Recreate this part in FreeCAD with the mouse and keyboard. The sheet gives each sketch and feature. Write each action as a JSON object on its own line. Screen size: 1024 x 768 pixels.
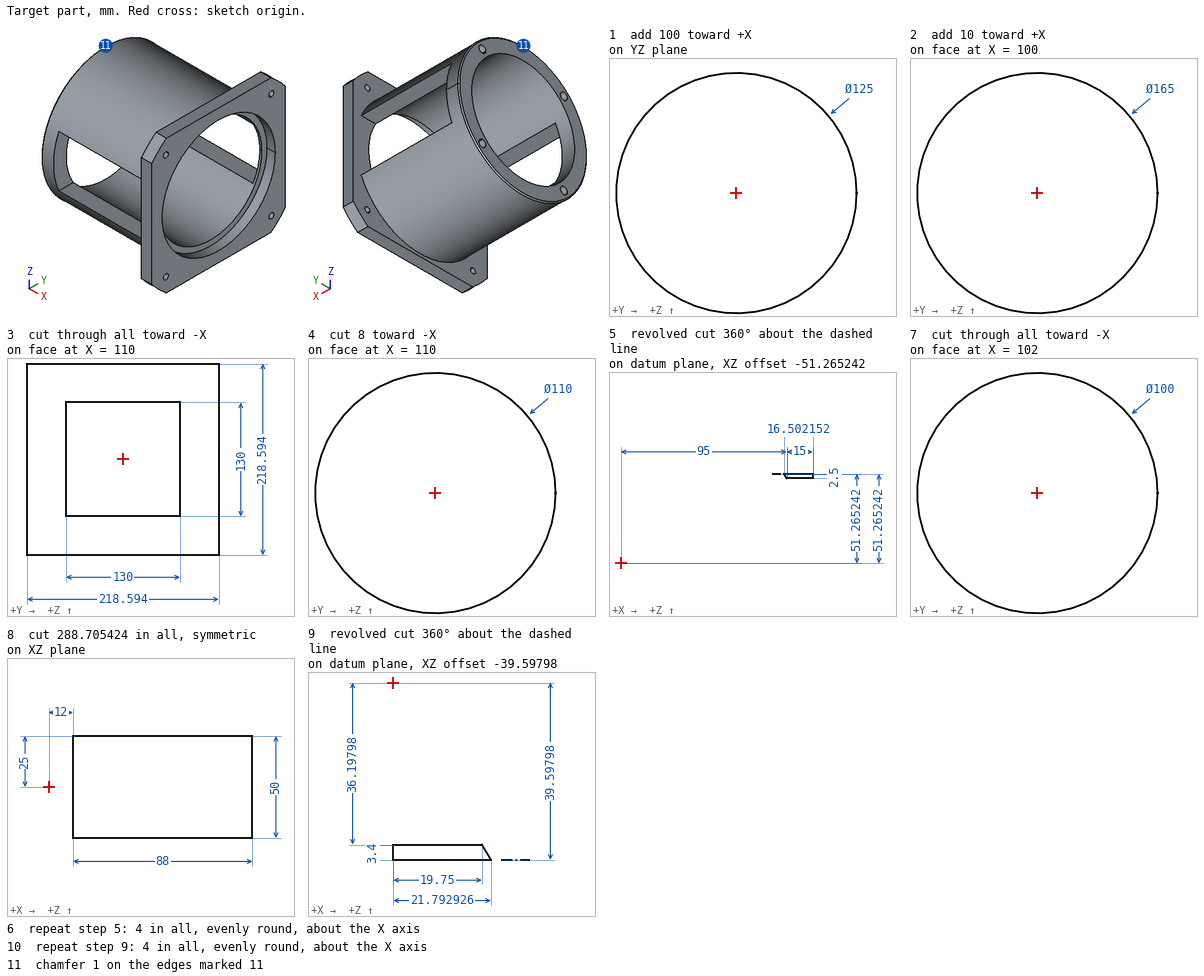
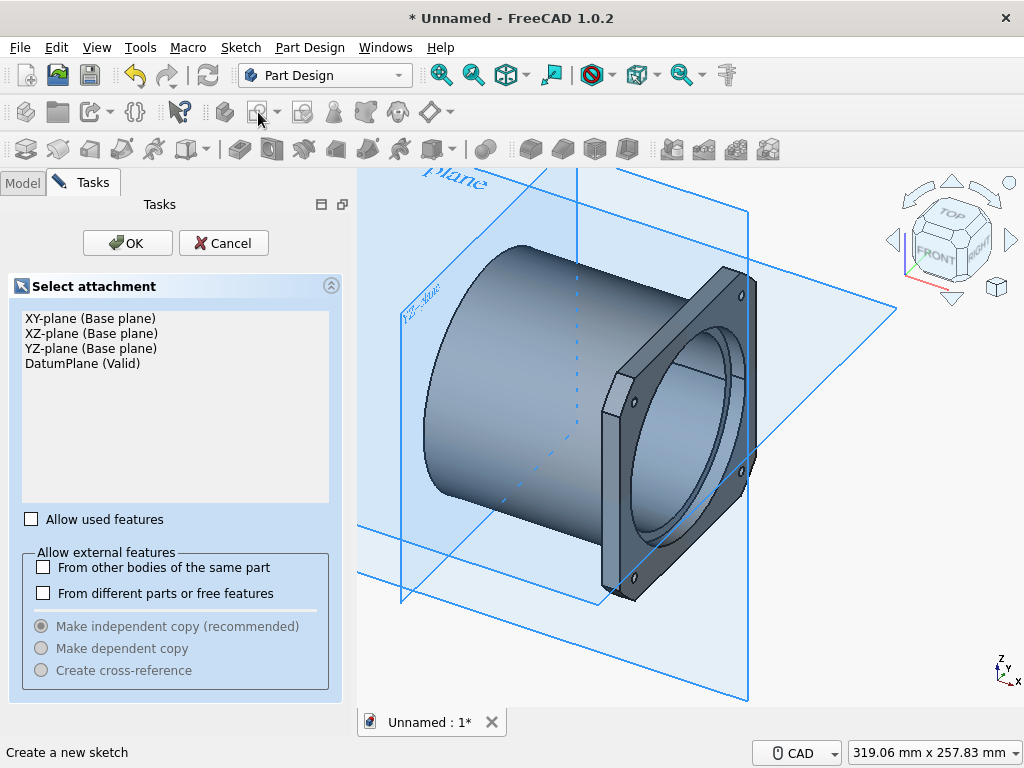
{"action": "left_click", "coordinate": [82, 334]}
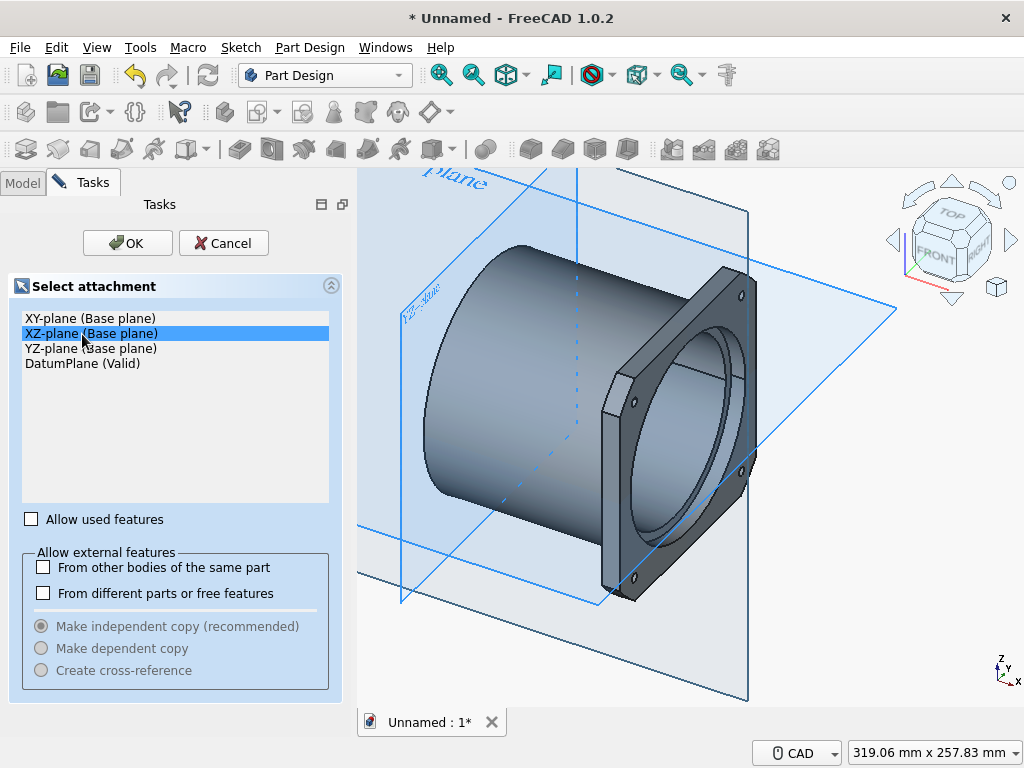
{"action": "left_click", "coordinate": [128, 243]}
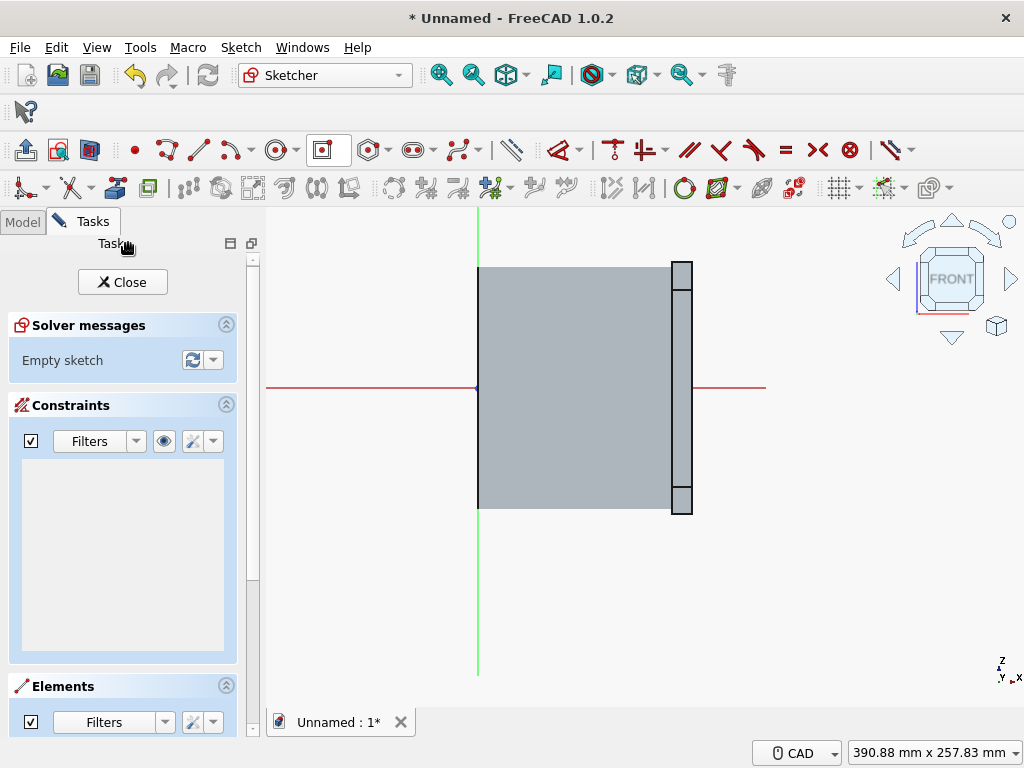
{"action": "left_click", "coordinate": [90, 150]}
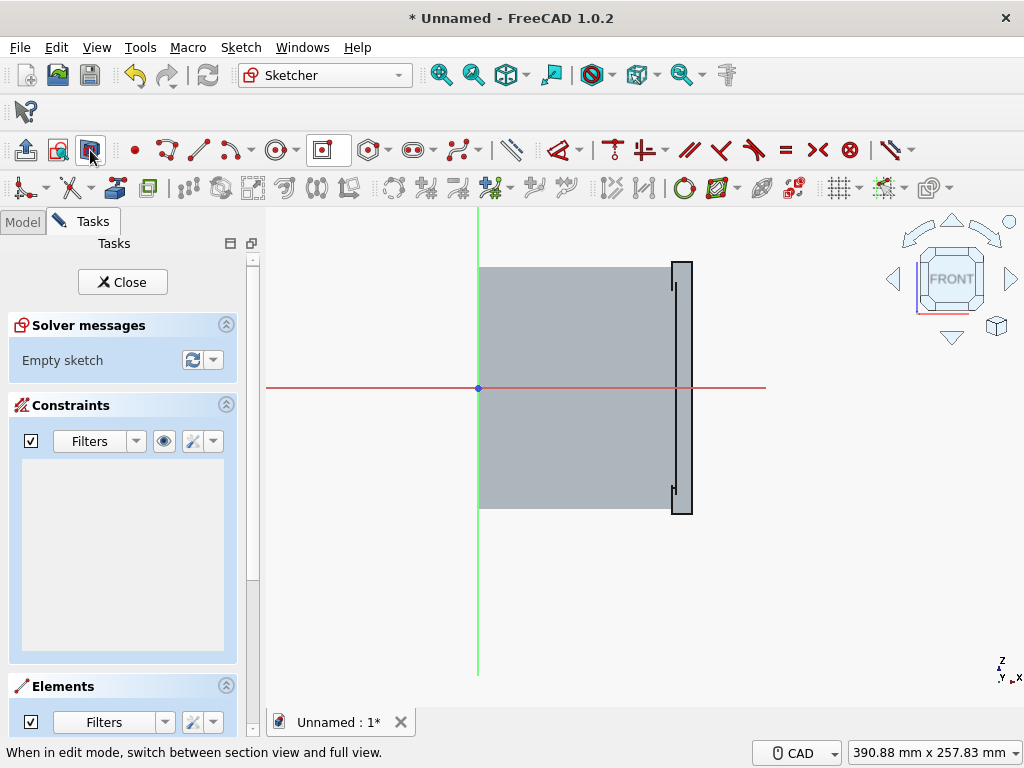
{"action": "scroll", "coordinate": [574, 332], "scroll_direction": "up", "scroll_amount": 4}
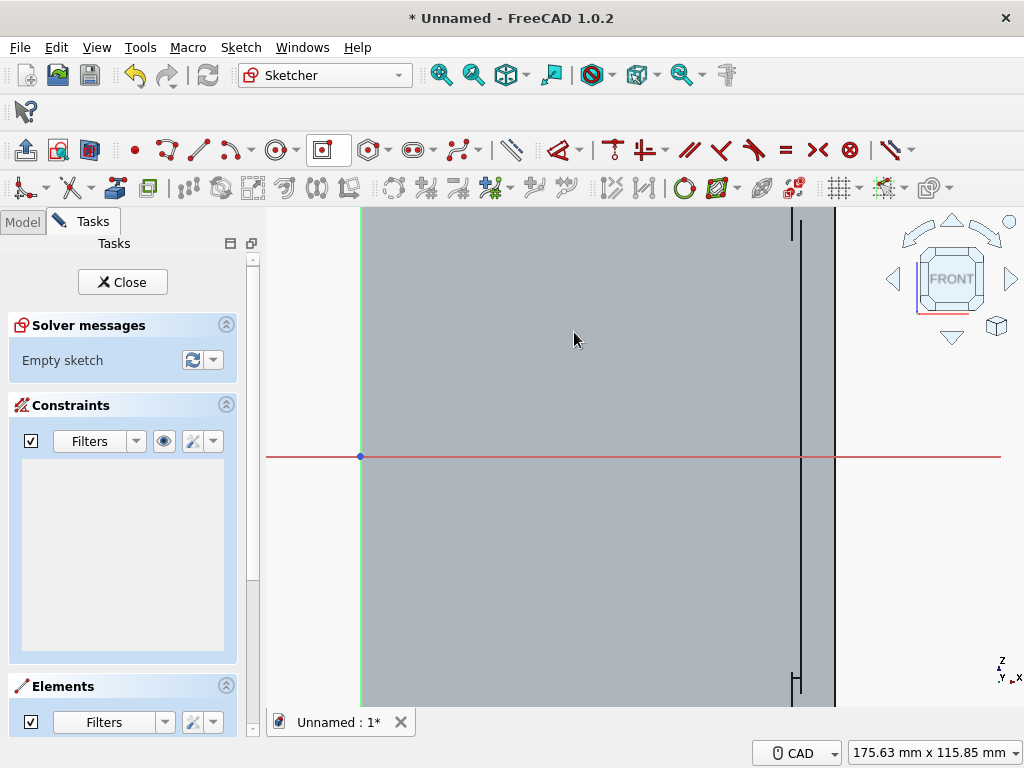
{"action": "key", "text": "g r"}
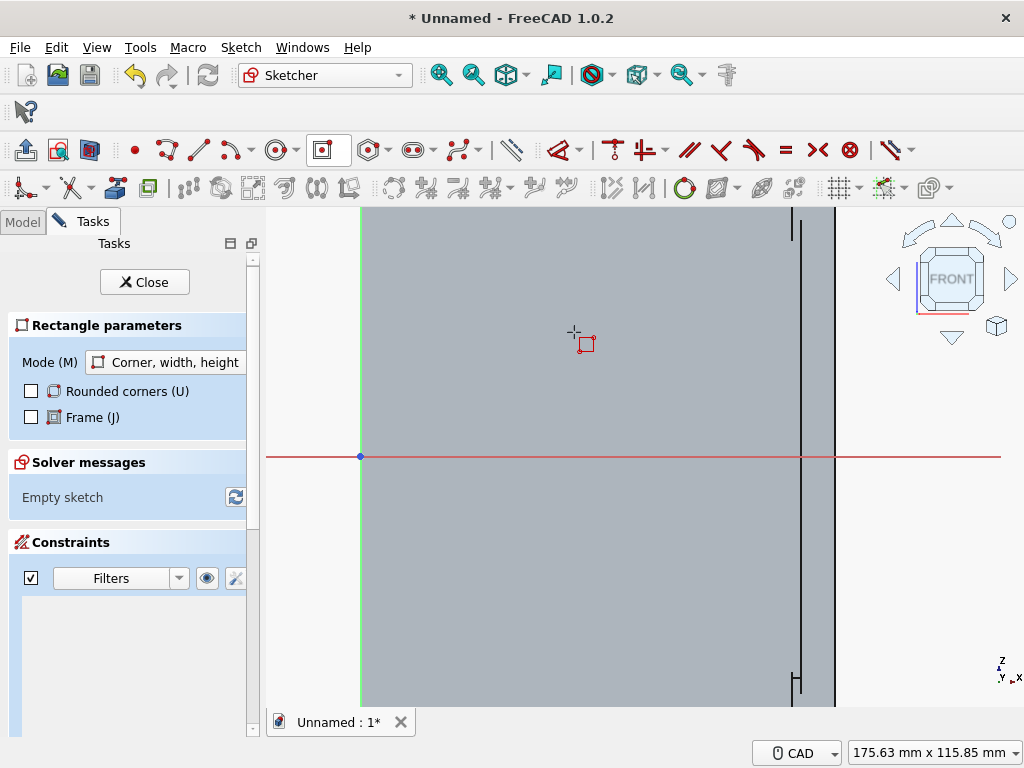
{"action": "left_click", "coordinate": [412, 349]}
{"action": "mouse_move", "coordinate": [792, 565]}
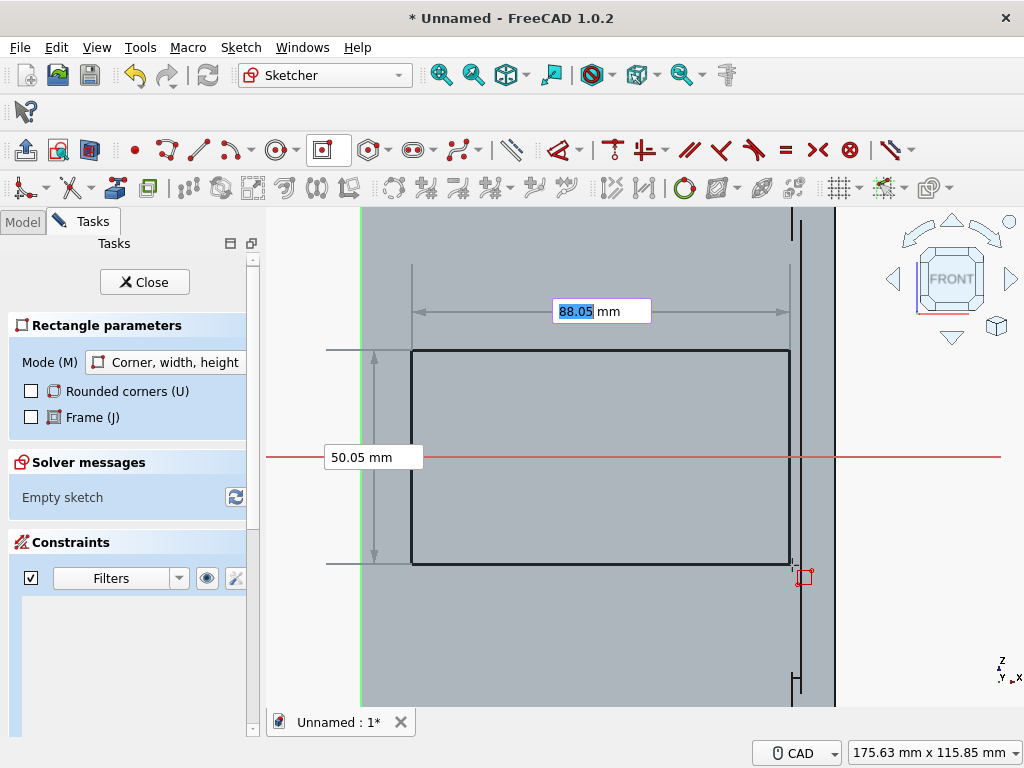
{"action": "type", "text": "88"}
{"action": "key", "text": "Tab"}
{"action": "type", "text": "50"}
{"action": "key", "text": "Return"}
{"action": "key", "text": "Escape"}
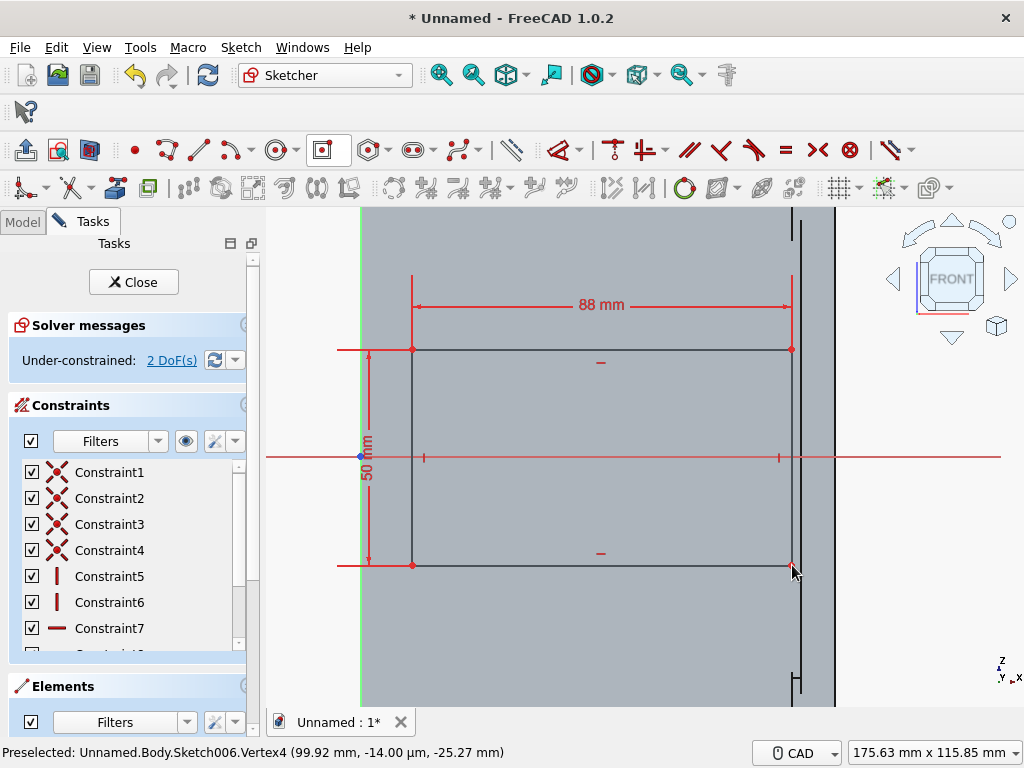
{"action": "left_click", "coordinate": [558, 150]}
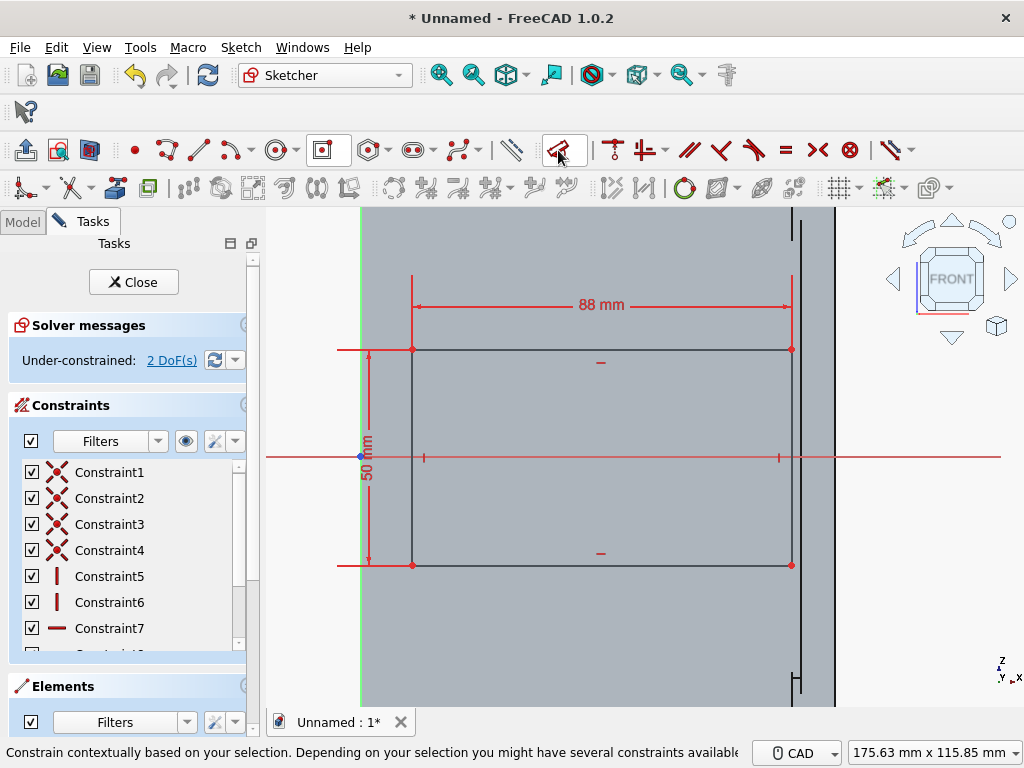
{"action": "left_click", "coordinate": [412, 350]}
{"action": "left_click", "coordinate": [386, 316]}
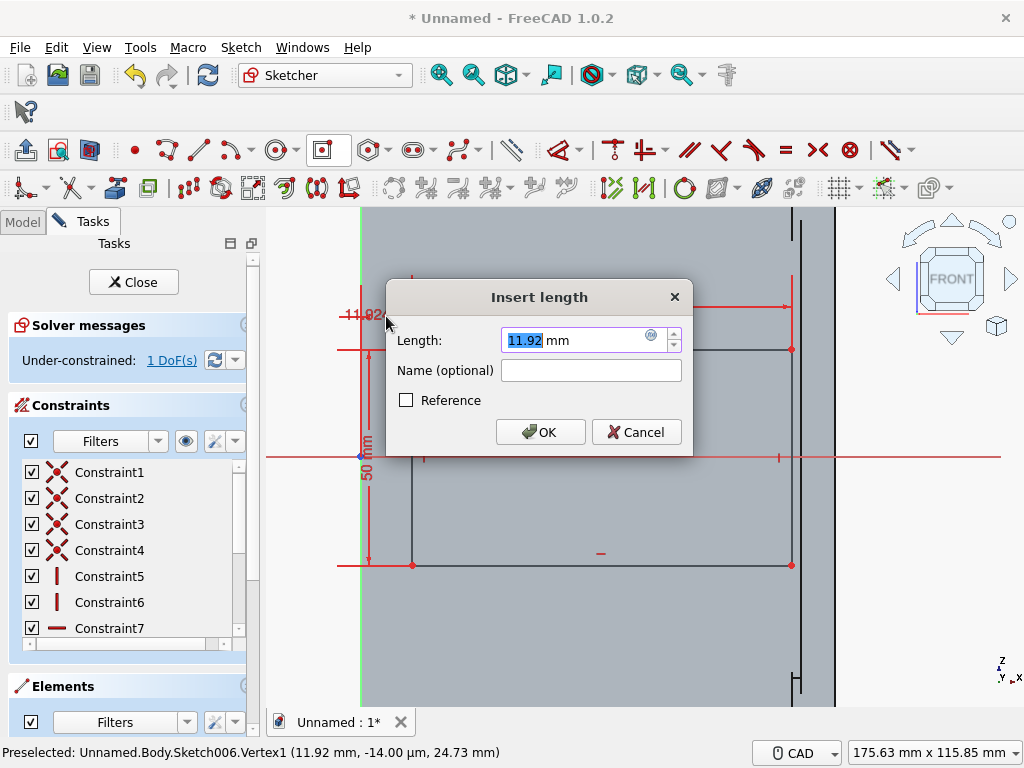
{"action": "type", "text": "12"}
{"action": "key", "text": "Return"}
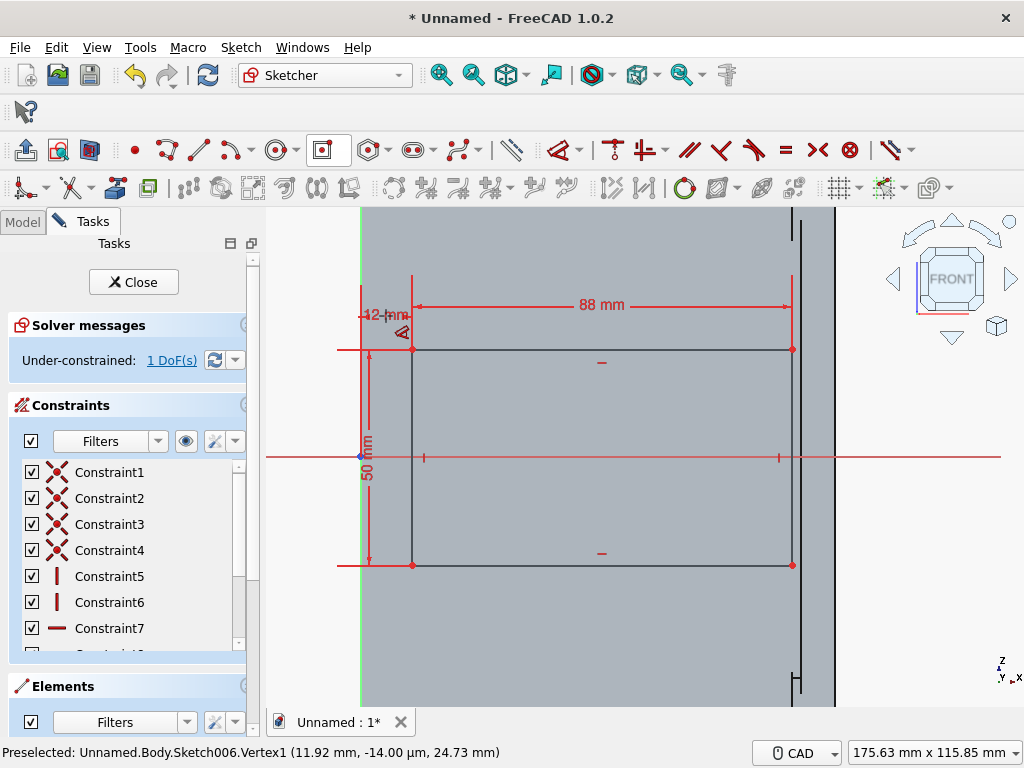
{"action": "left_click", "coordinate": [412, 350]}
{"action": "left_click", "coordinate": [327, 403]}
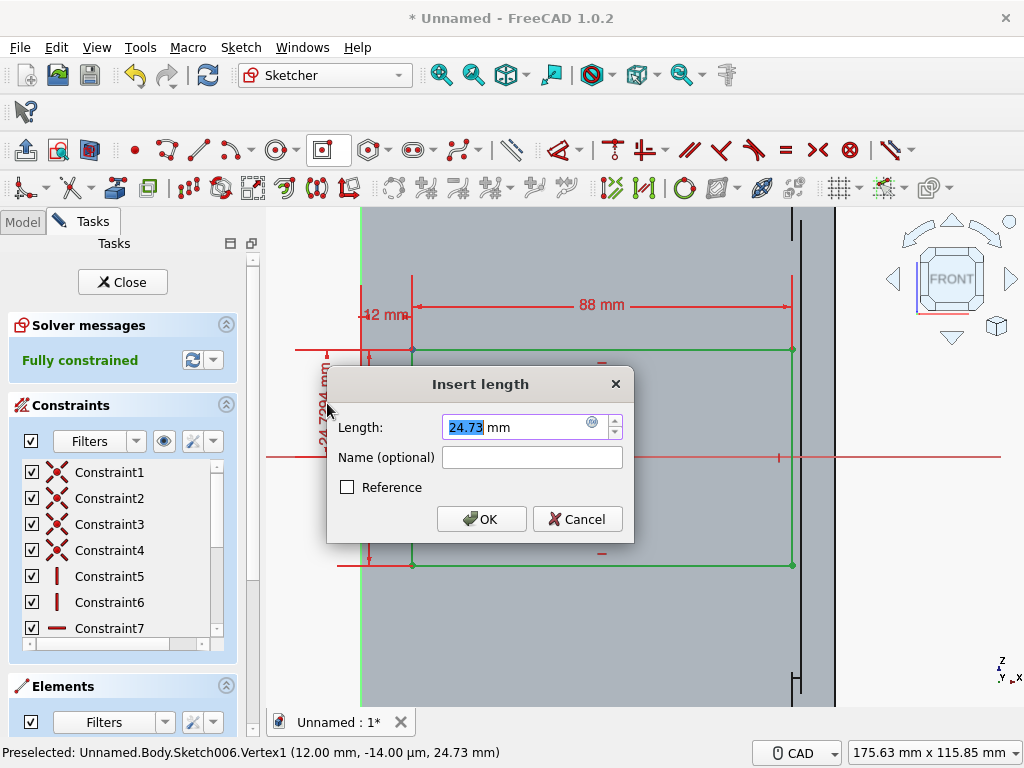
{"action": "type", "text": "25"}
{"action": "key", "text": "Return"}
{"action": "key", "text": "Escape"}